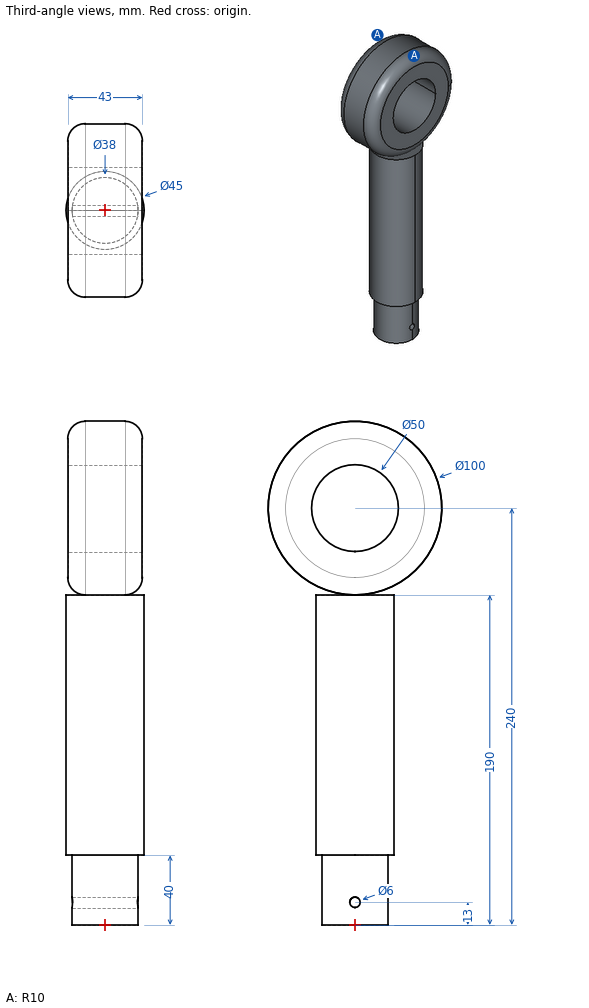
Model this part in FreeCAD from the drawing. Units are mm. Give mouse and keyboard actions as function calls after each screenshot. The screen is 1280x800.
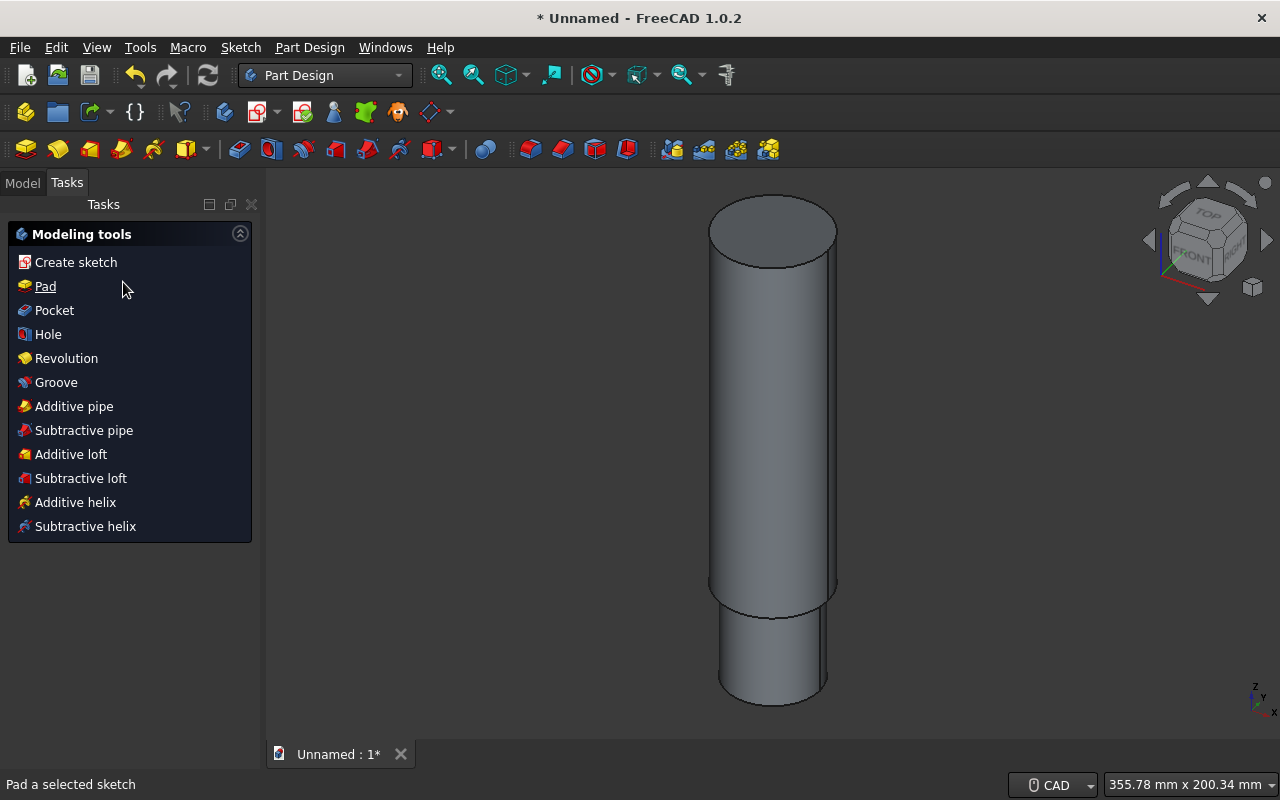
click(240, 150)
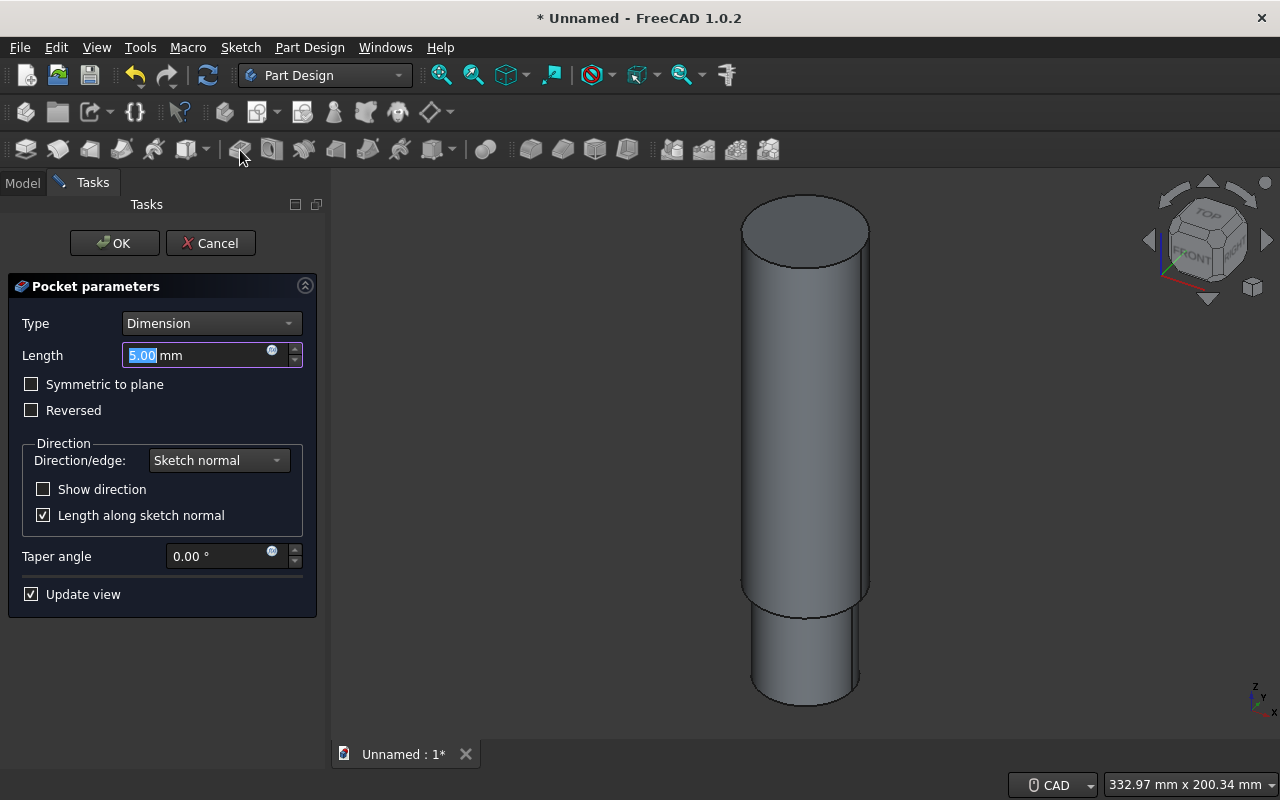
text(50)
key(Tab)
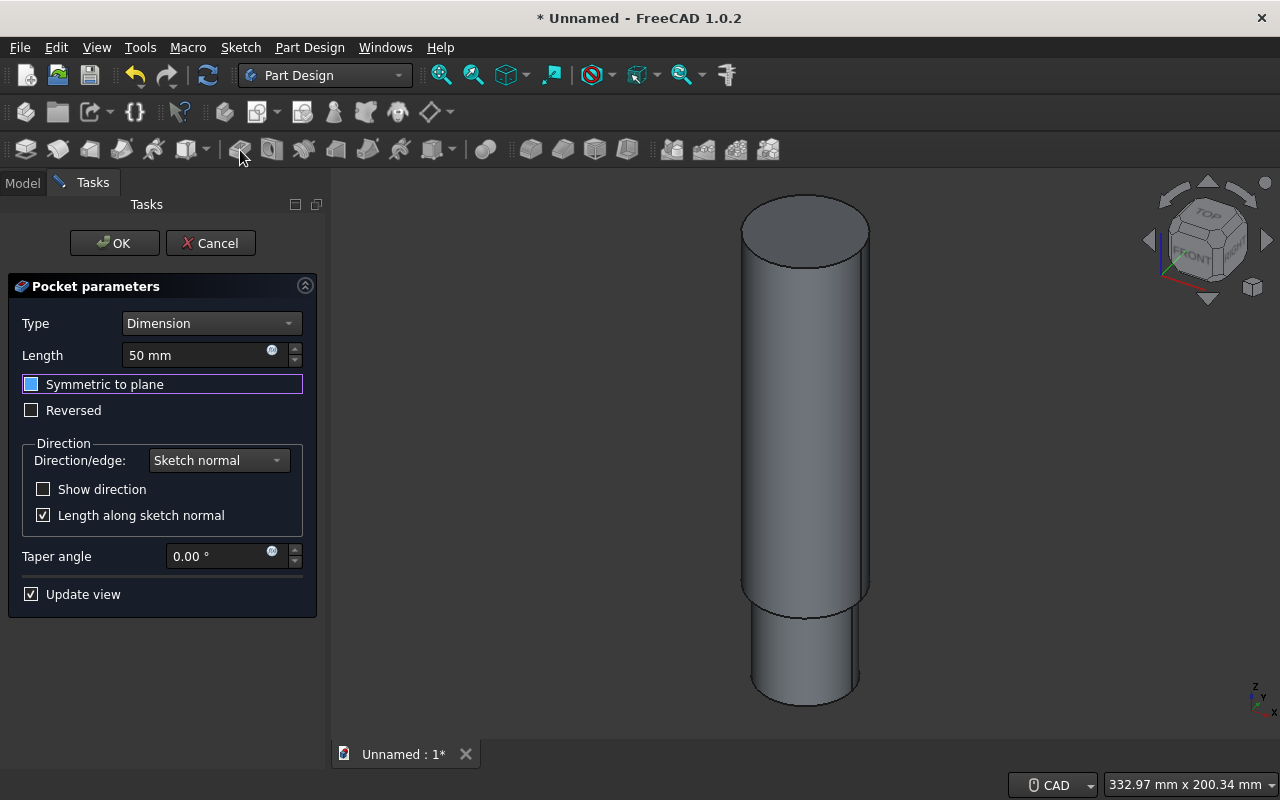
click(30, 384)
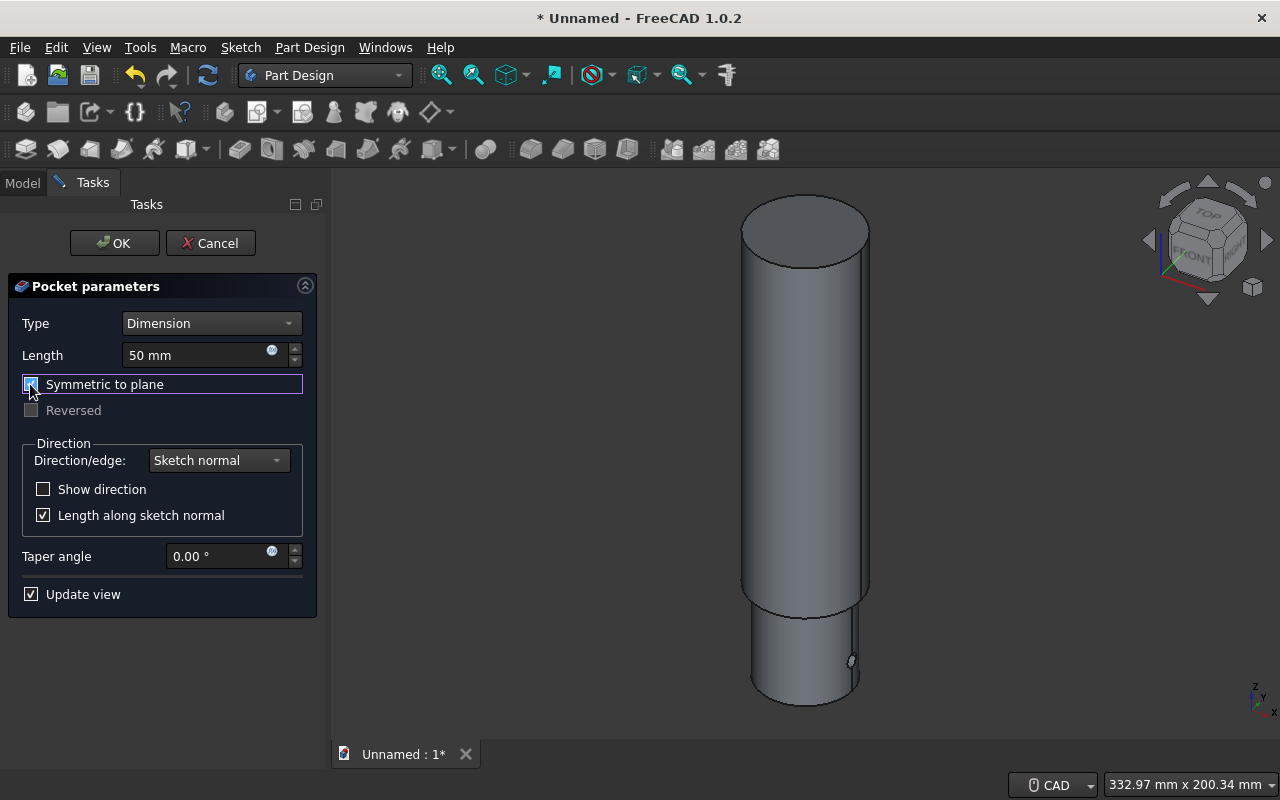
click(115, 243)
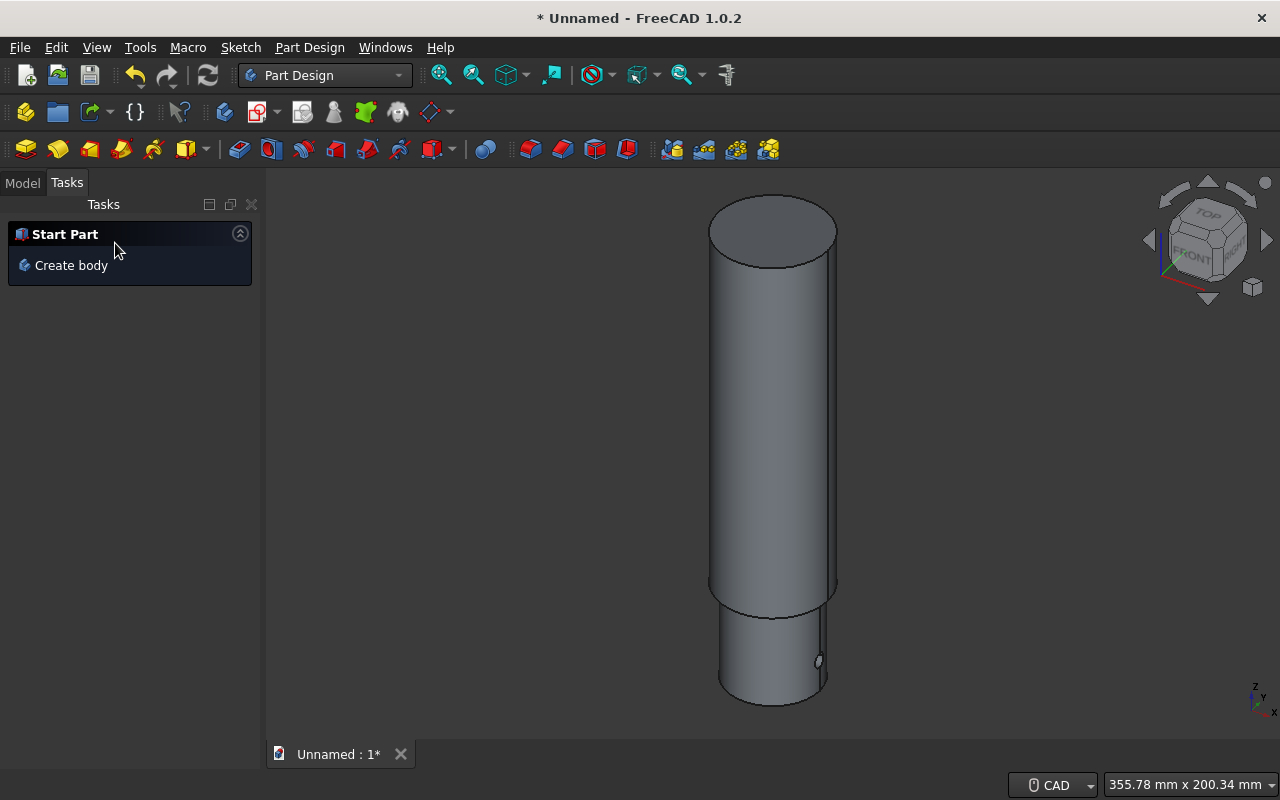
click(226, 112)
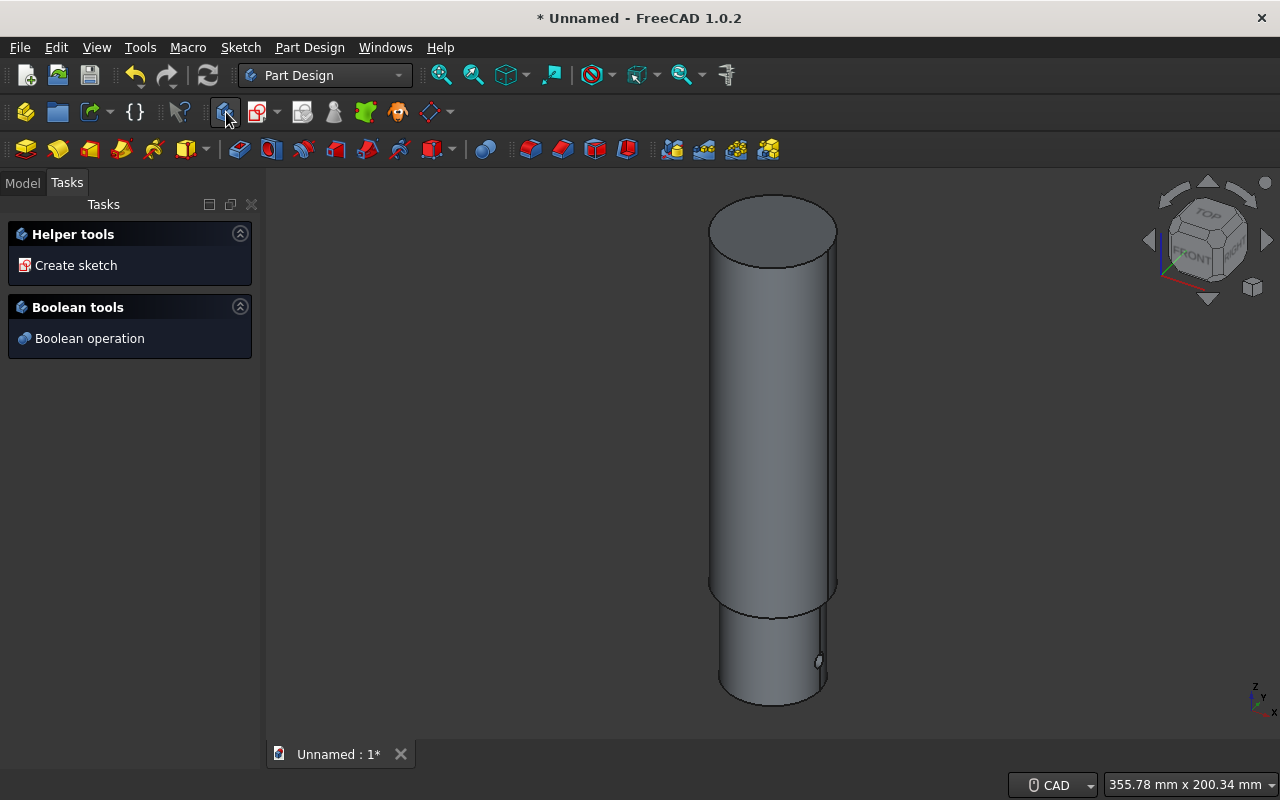
click(306, 699)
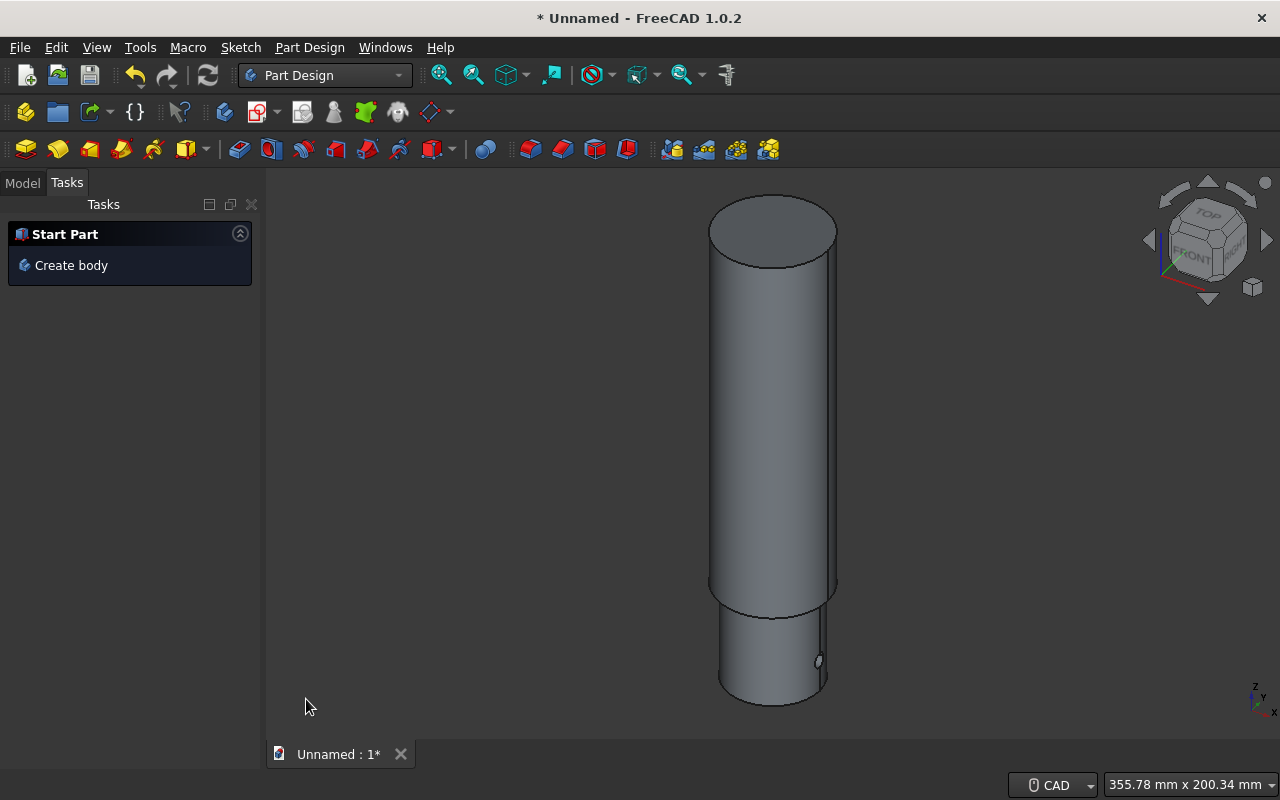
click(258, 112)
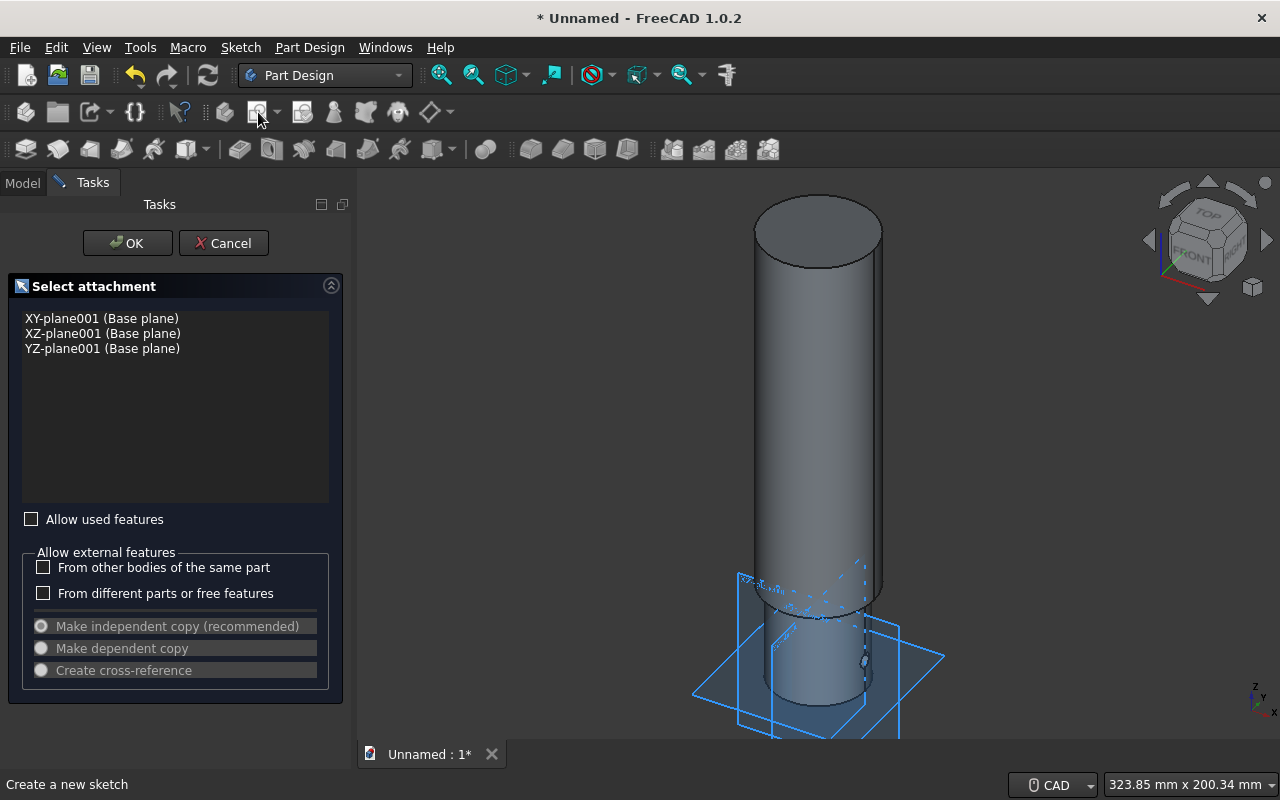
click(82, 348)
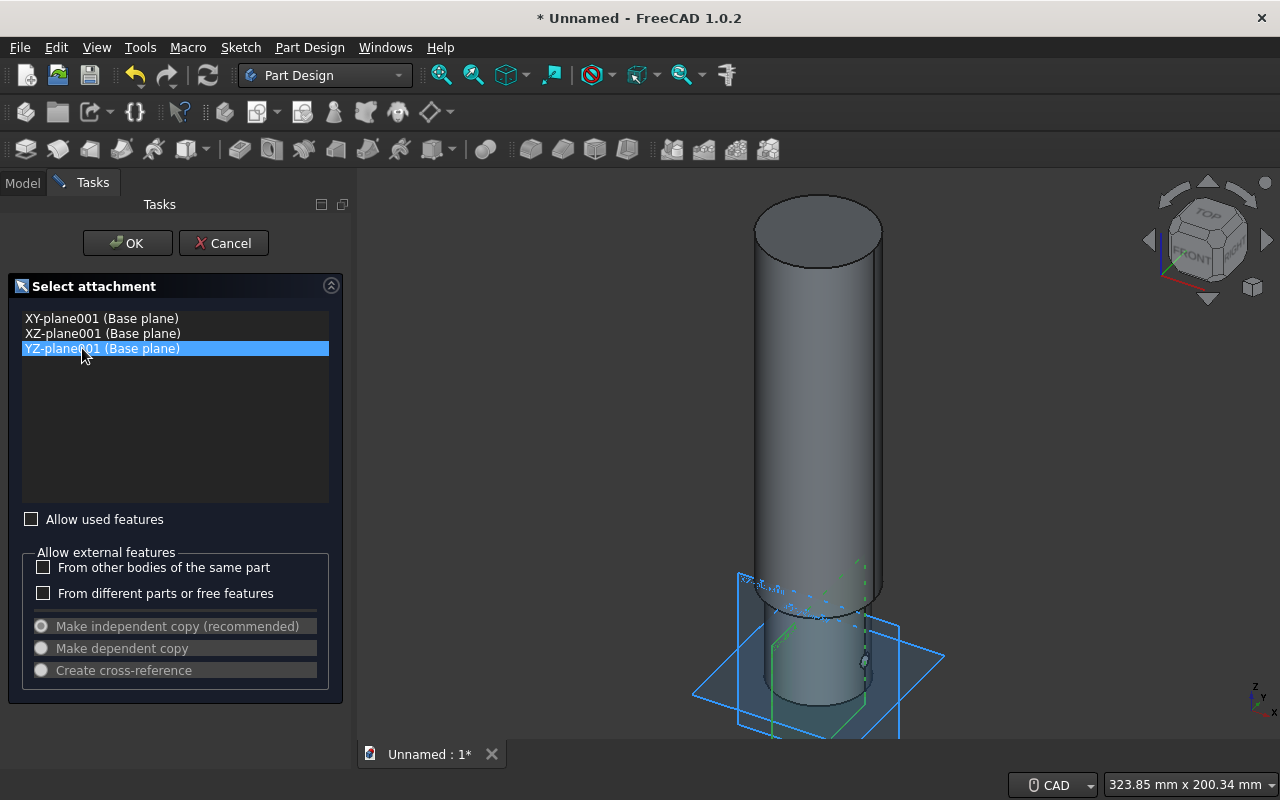
click(128, 243)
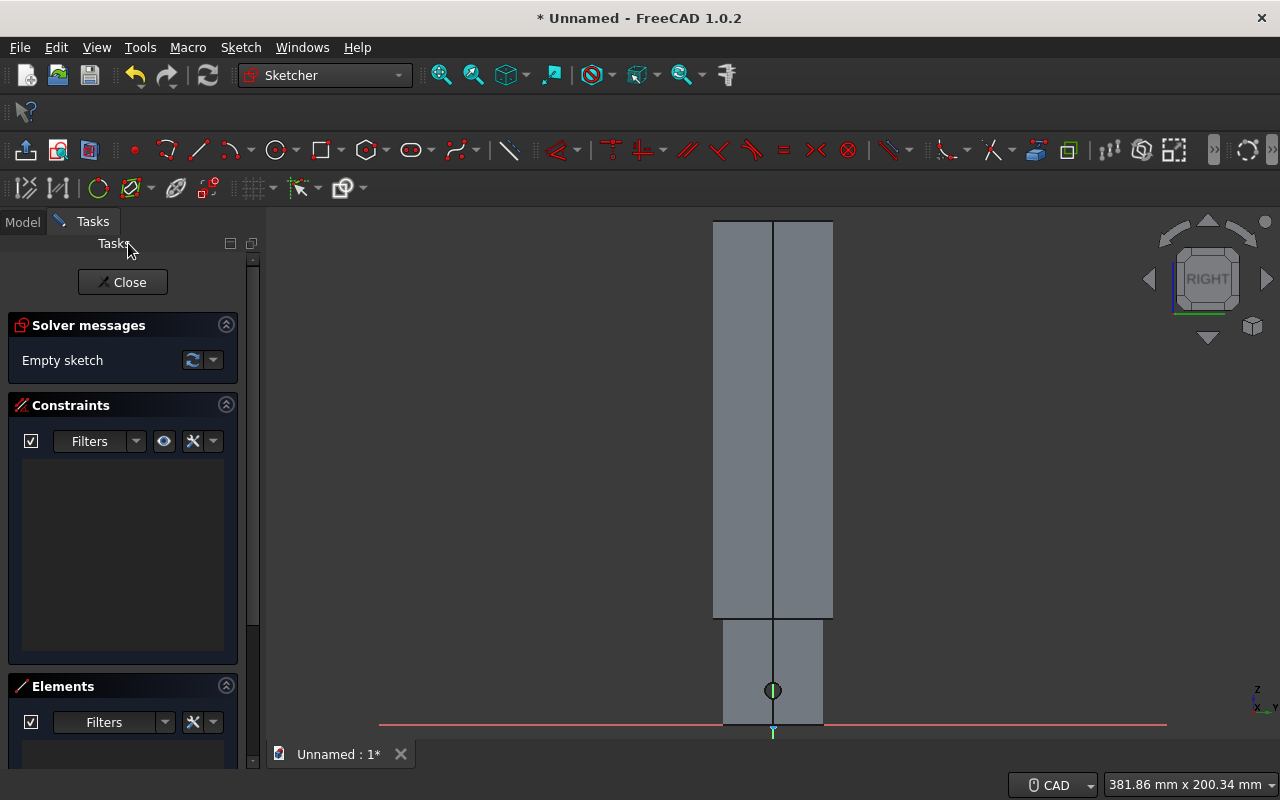
scroll(704, 473, down, 5)